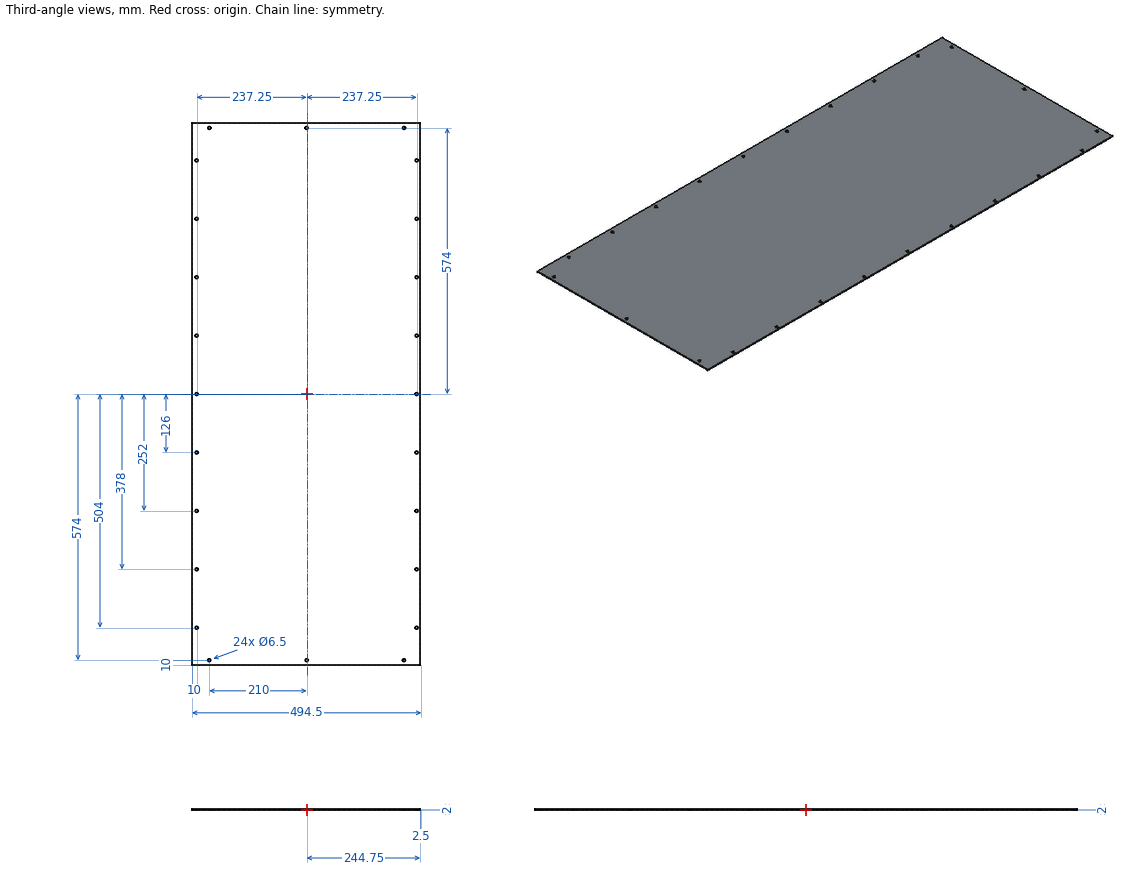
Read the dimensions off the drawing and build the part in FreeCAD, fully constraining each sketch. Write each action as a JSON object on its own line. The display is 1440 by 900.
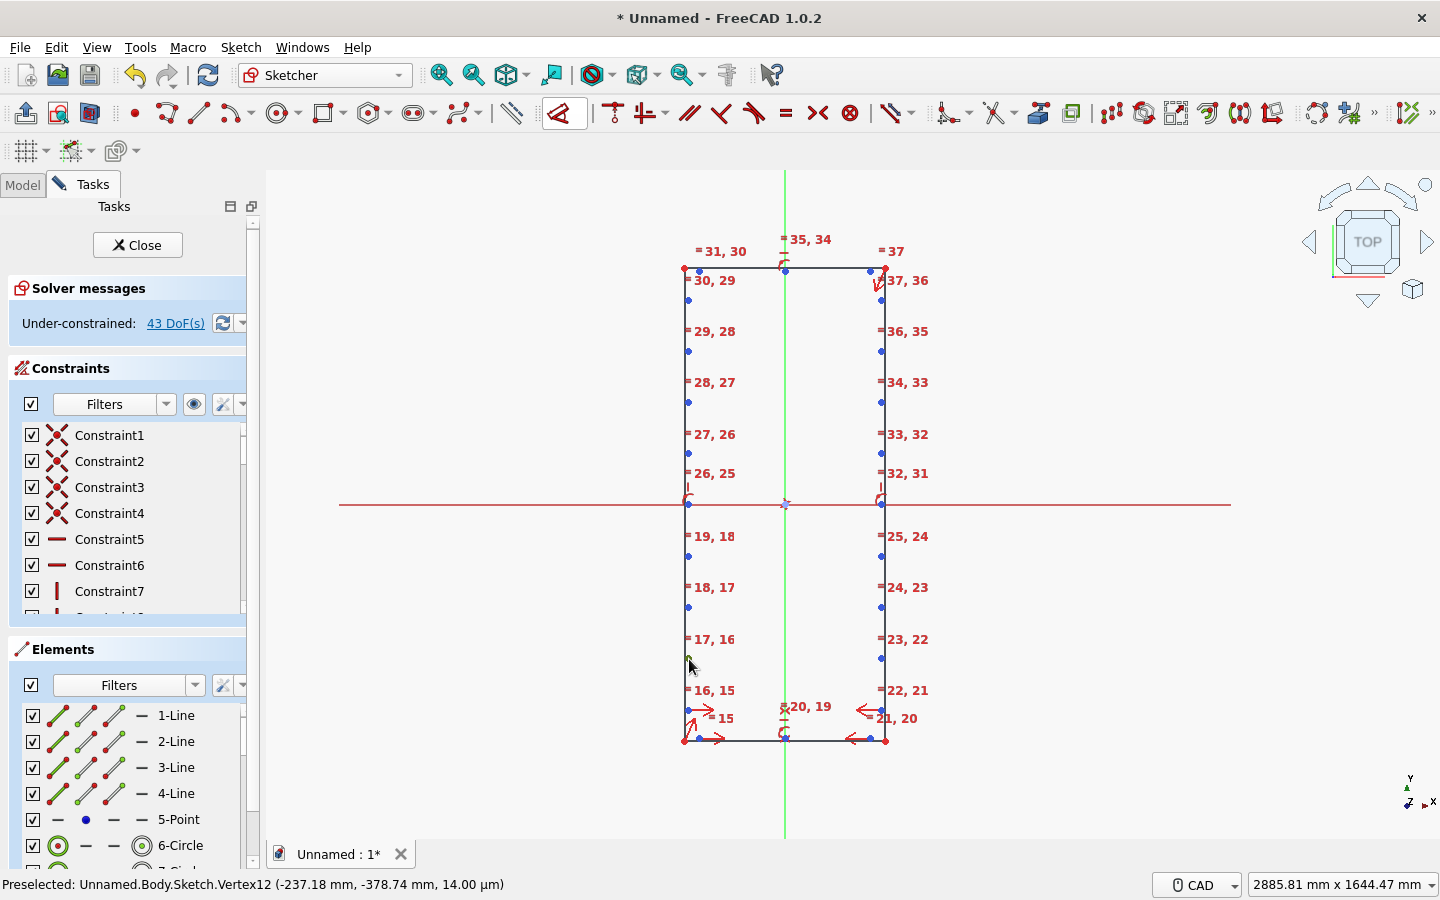
{"action": "left_click", "coordinate": [882, 659]}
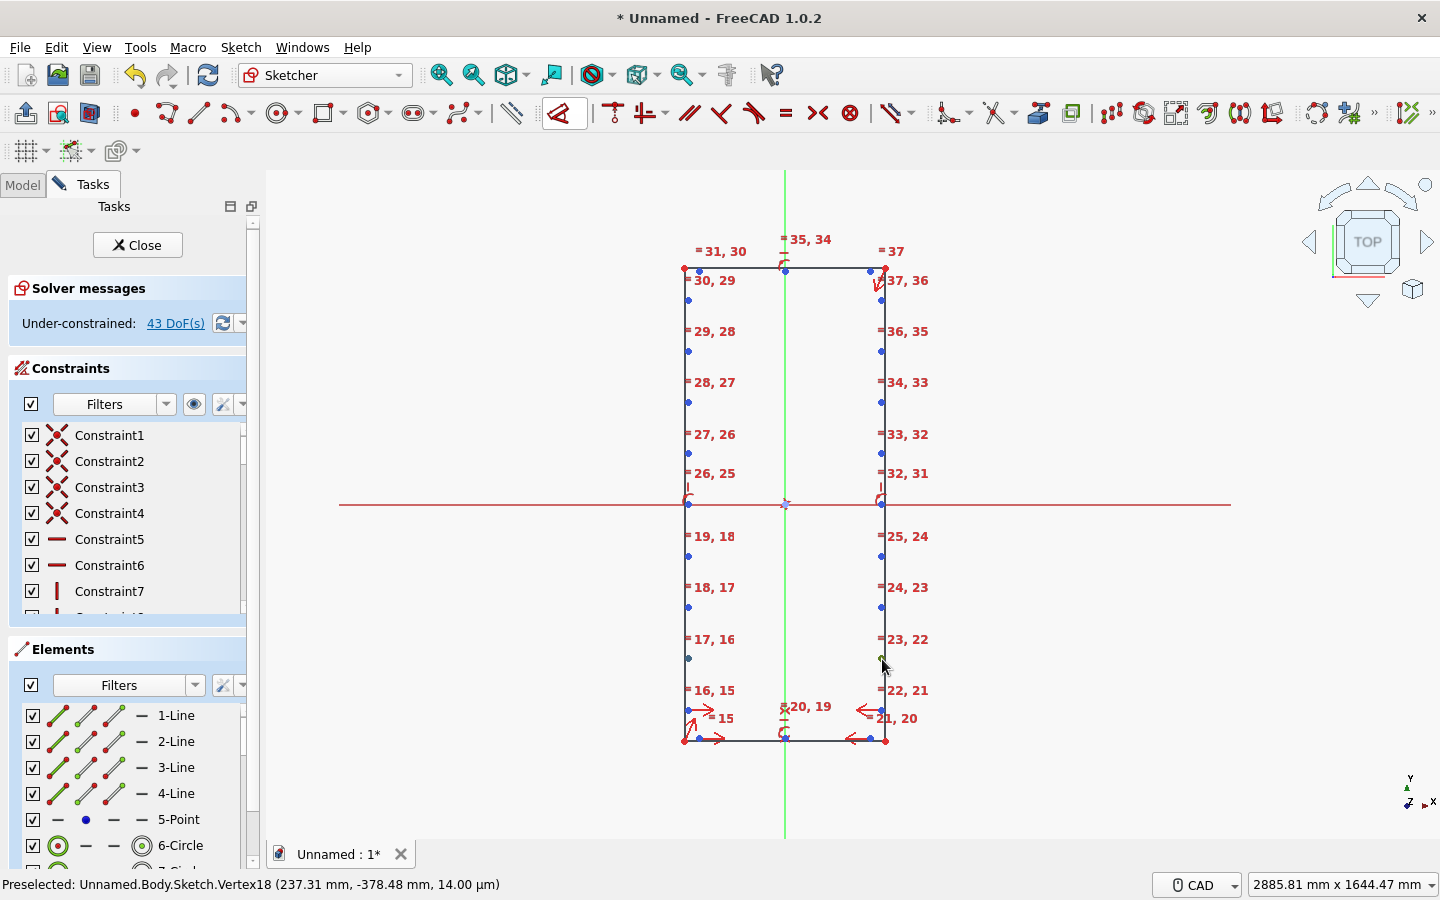
{"action": "left_click", "coordinate": [785, 680]}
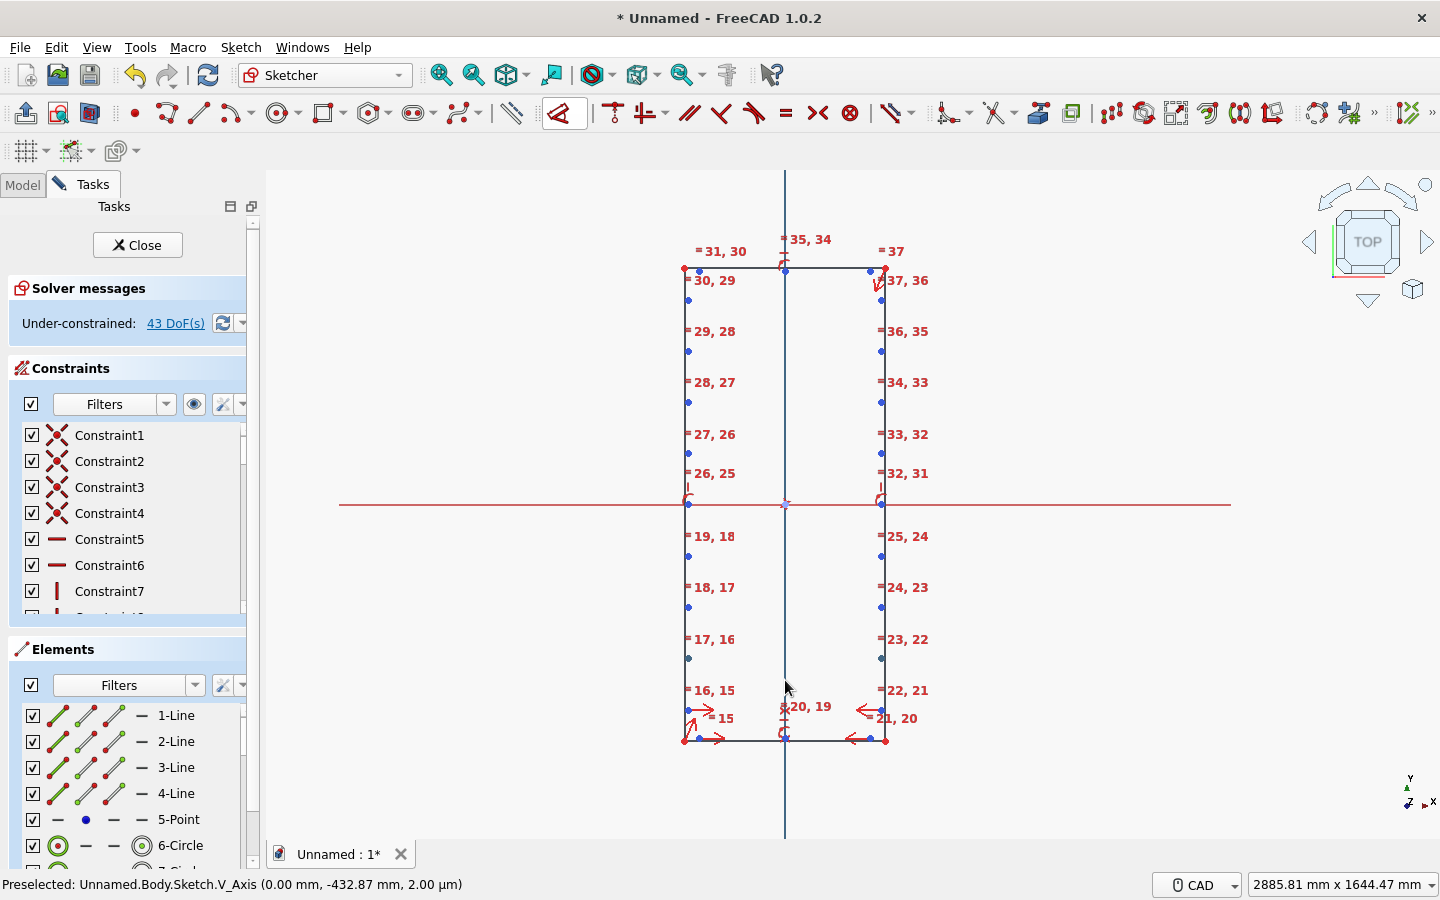
{"action": "key", "text": "s"}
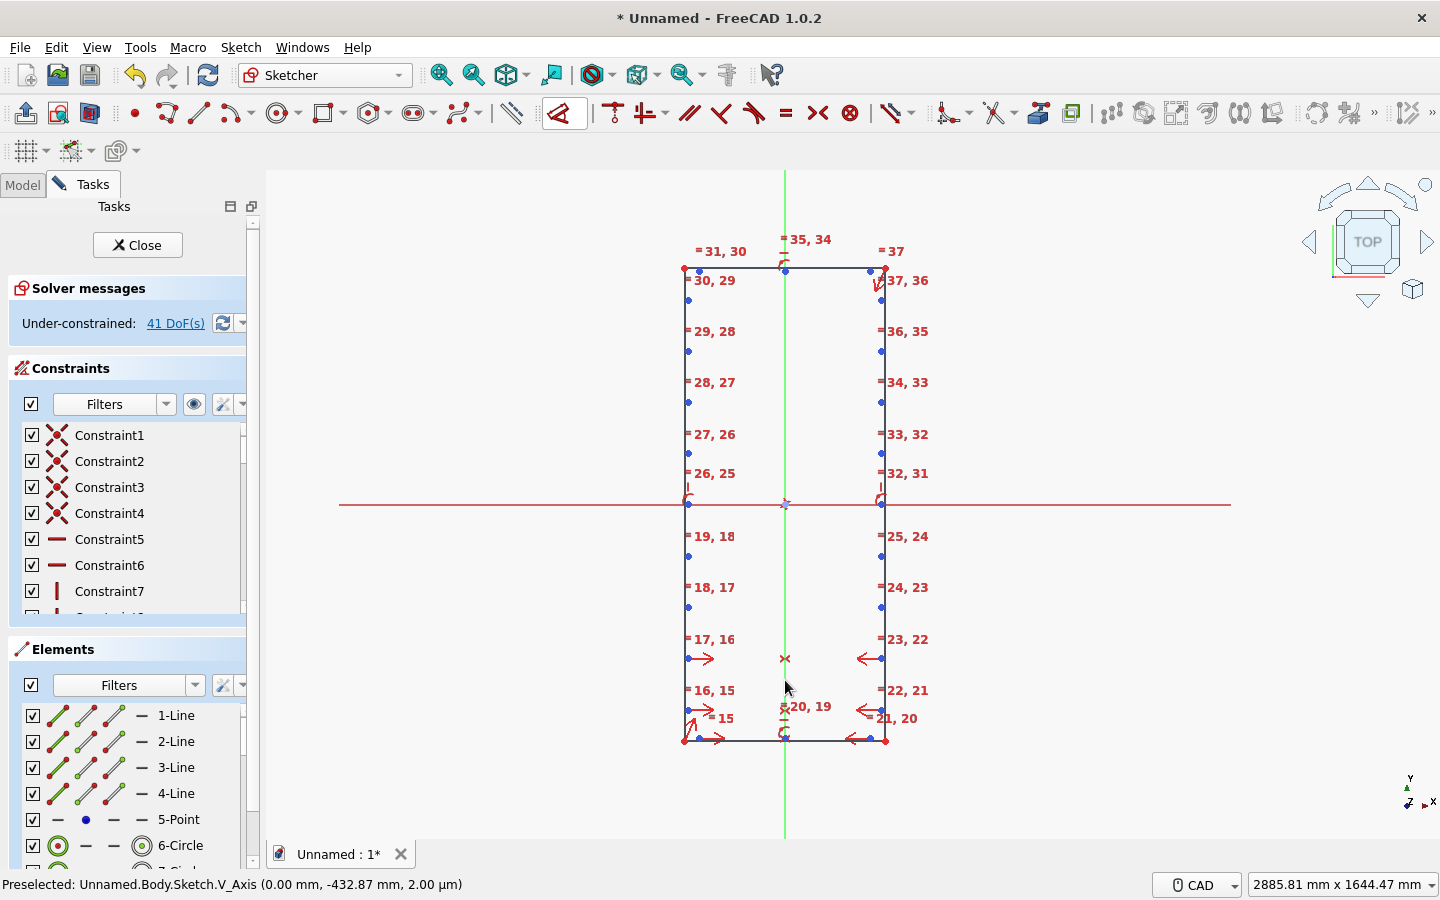
{"action": "left_click", "coordinate": [689, 608]}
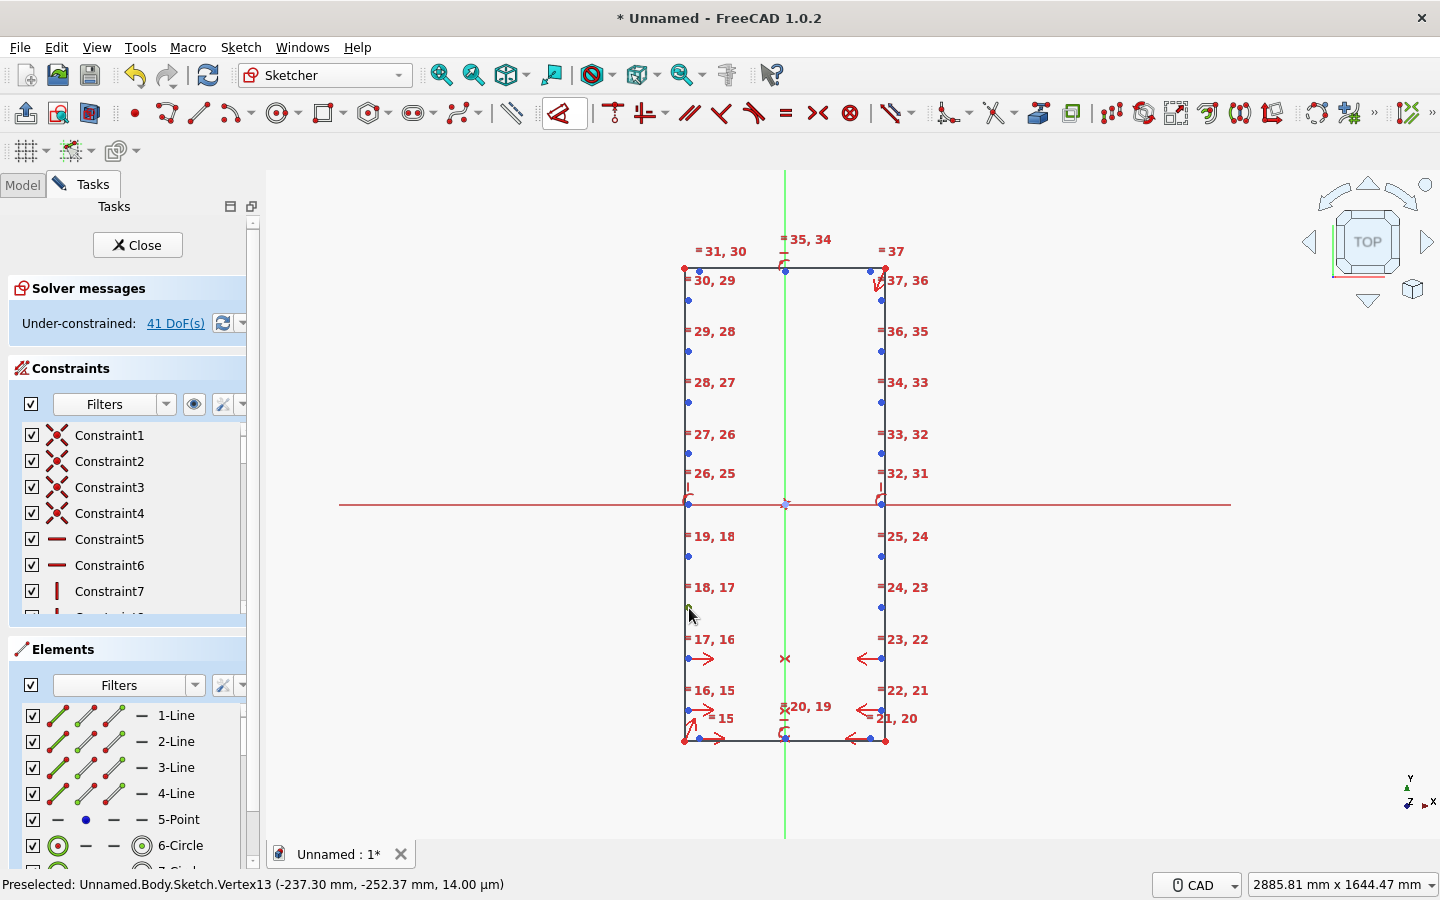
{"action": "left_click", "coordinate": [882, 608]}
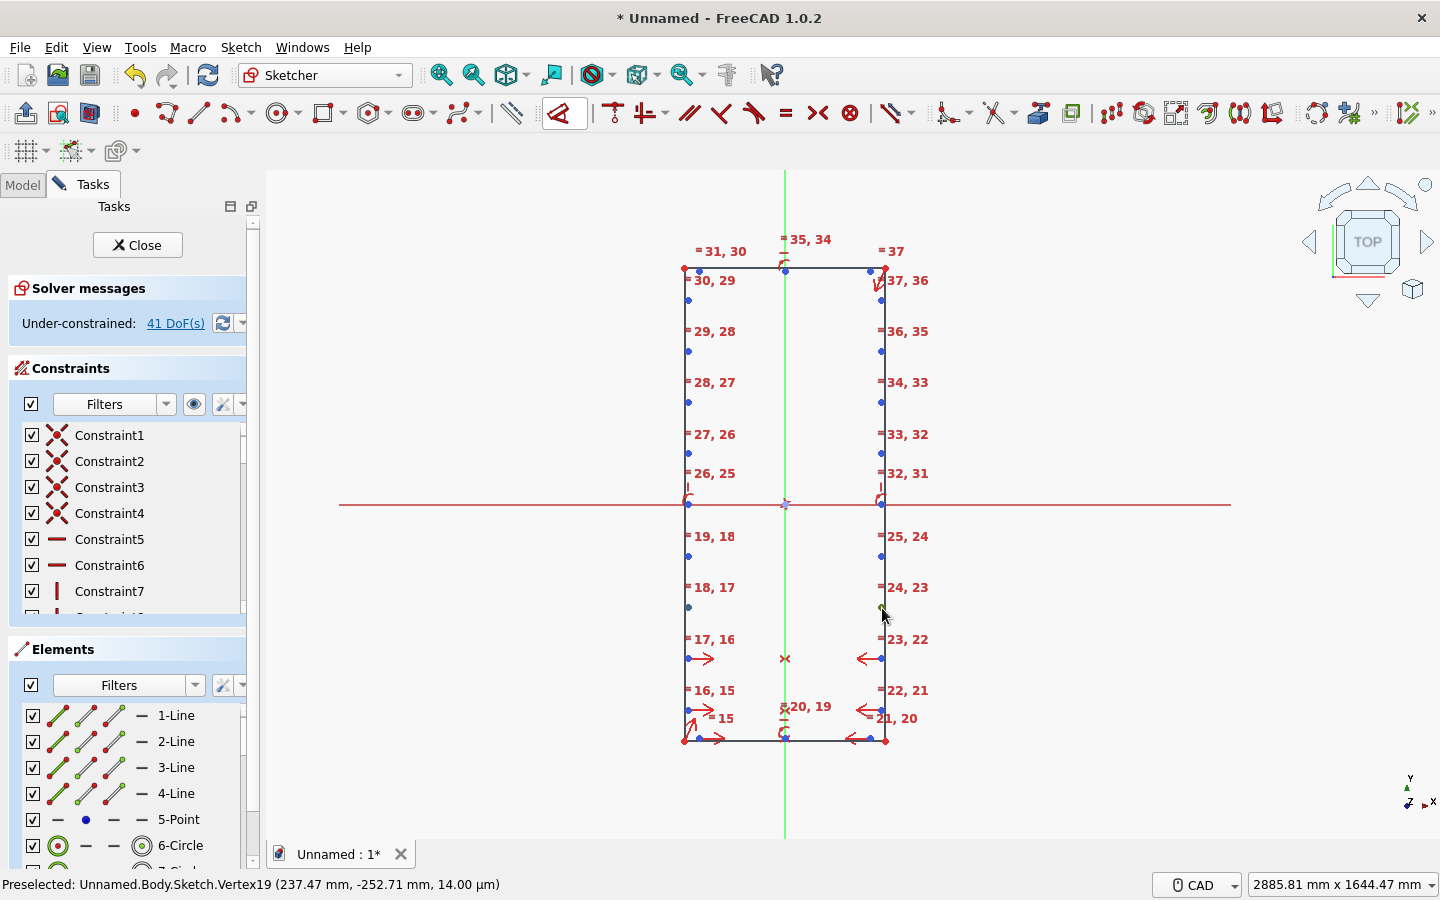
{"action": "left_click", "coordinate": [785, 680]}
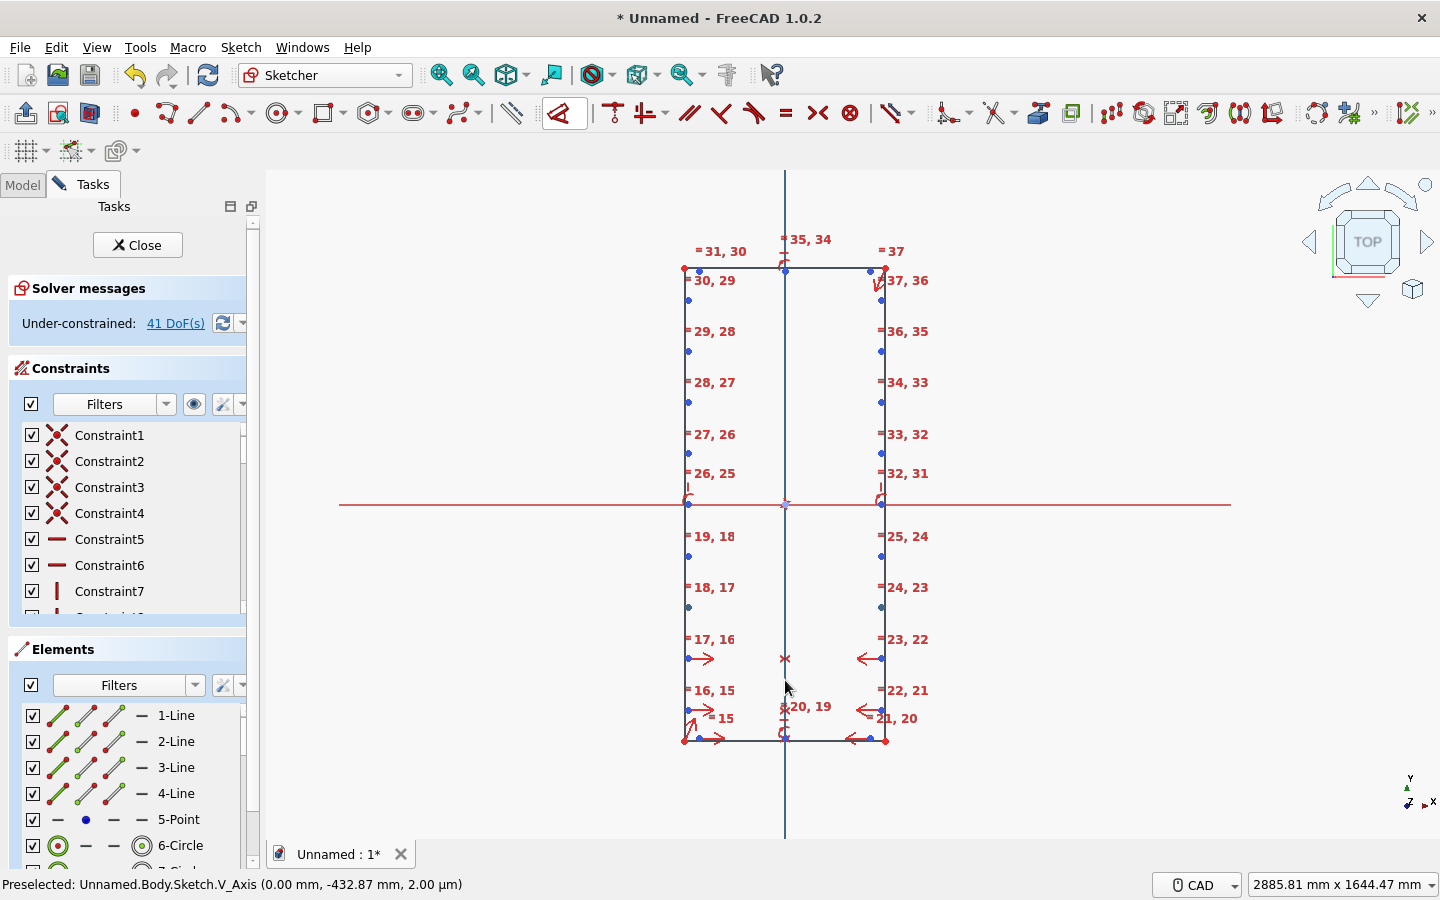
{"action": "key", "text": "s"}